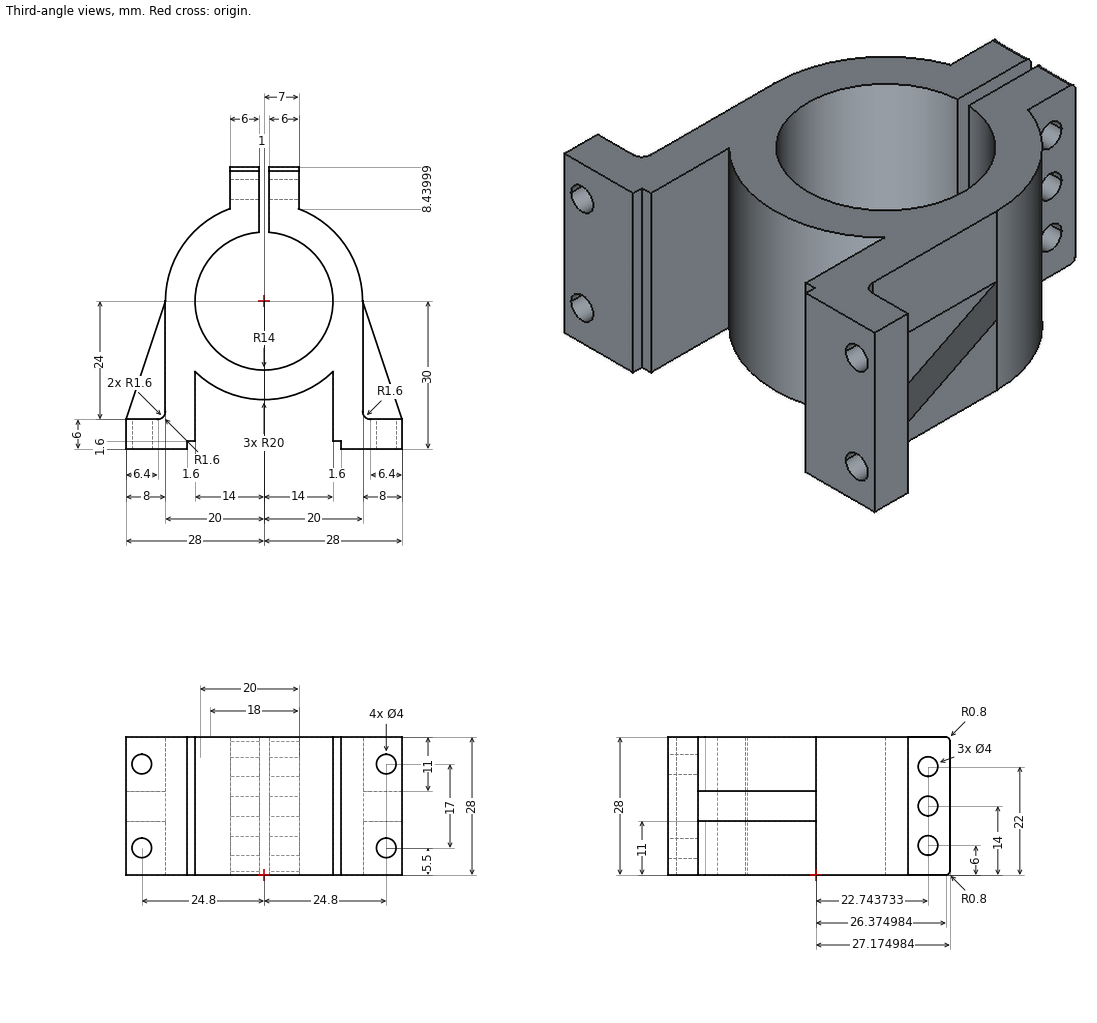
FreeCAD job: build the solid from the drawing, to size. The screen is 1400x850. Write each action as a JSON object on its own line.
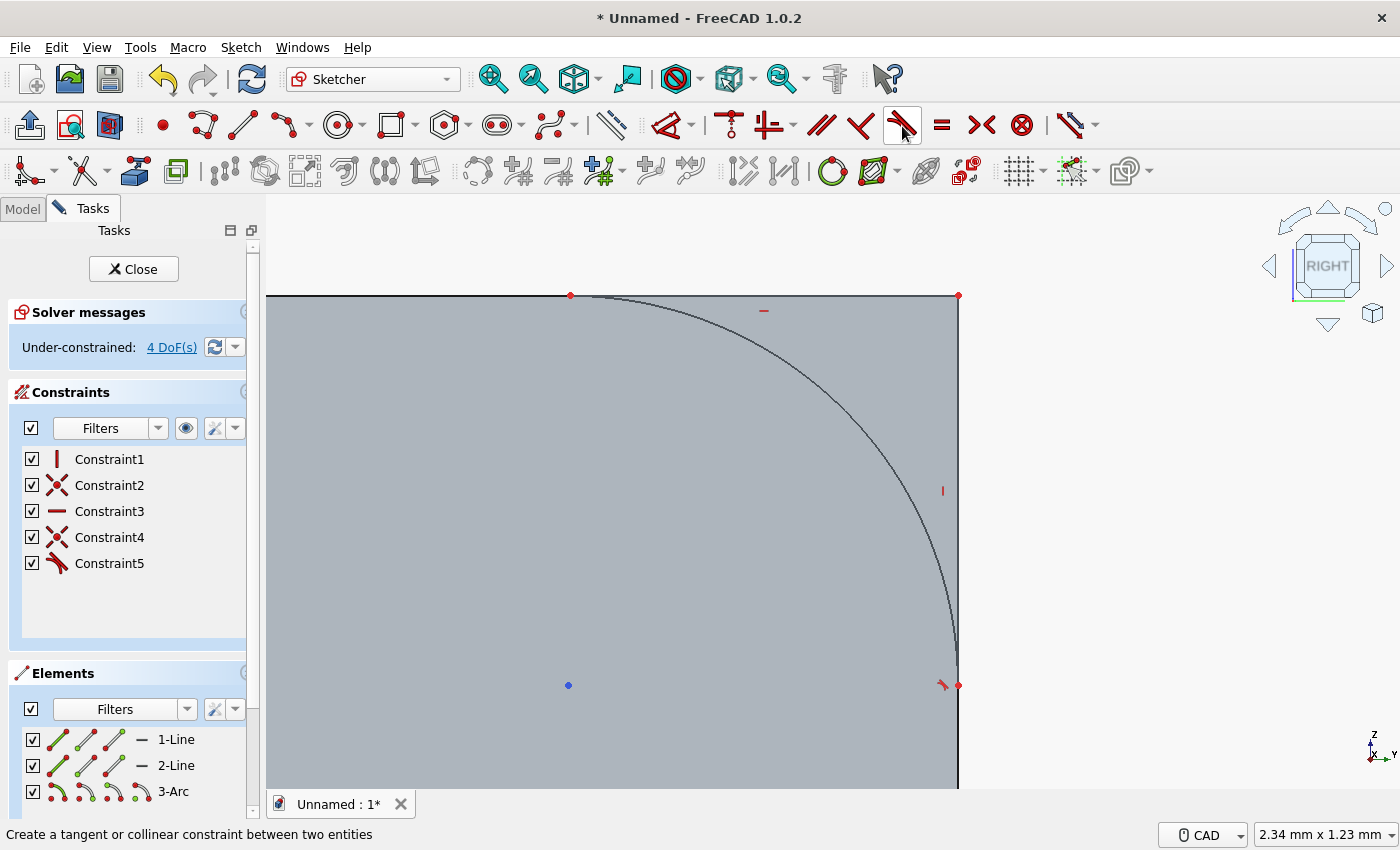
{"action": "left_click", "coordinate": [842, 296]}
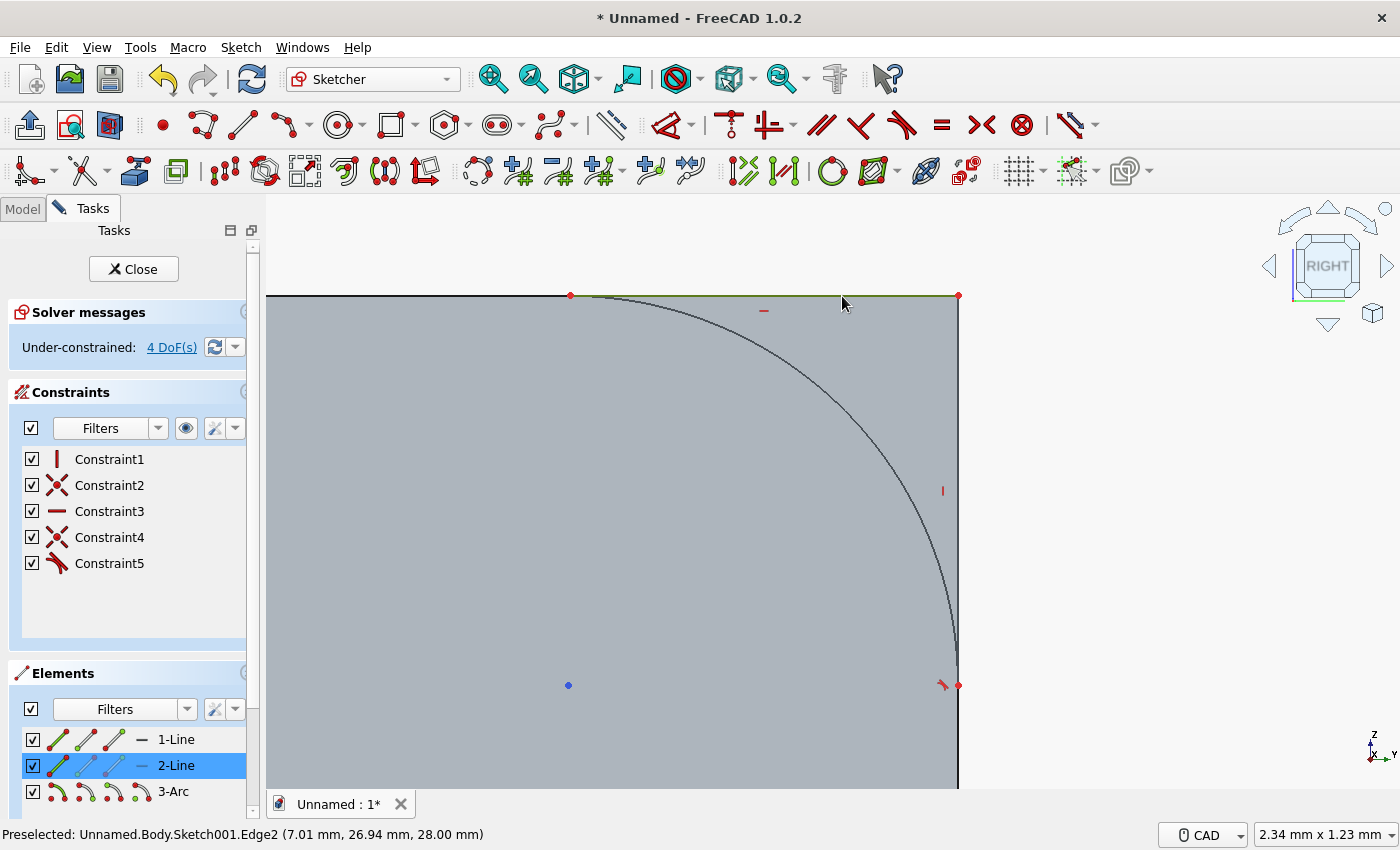
{"action": "left_click", "coordinate": [916, 509]}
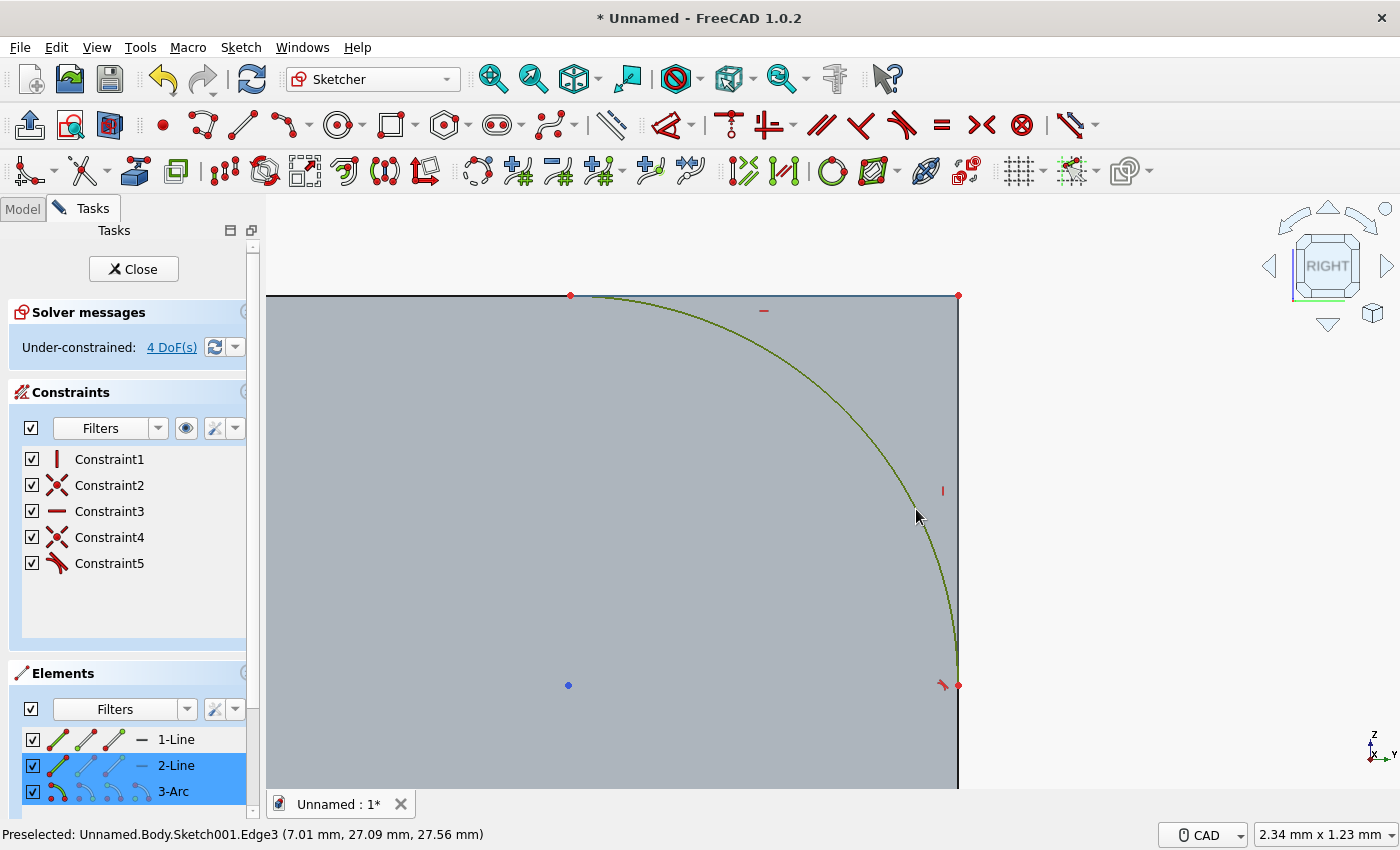
{"action": "left_click", "coordinate": [902, 126]}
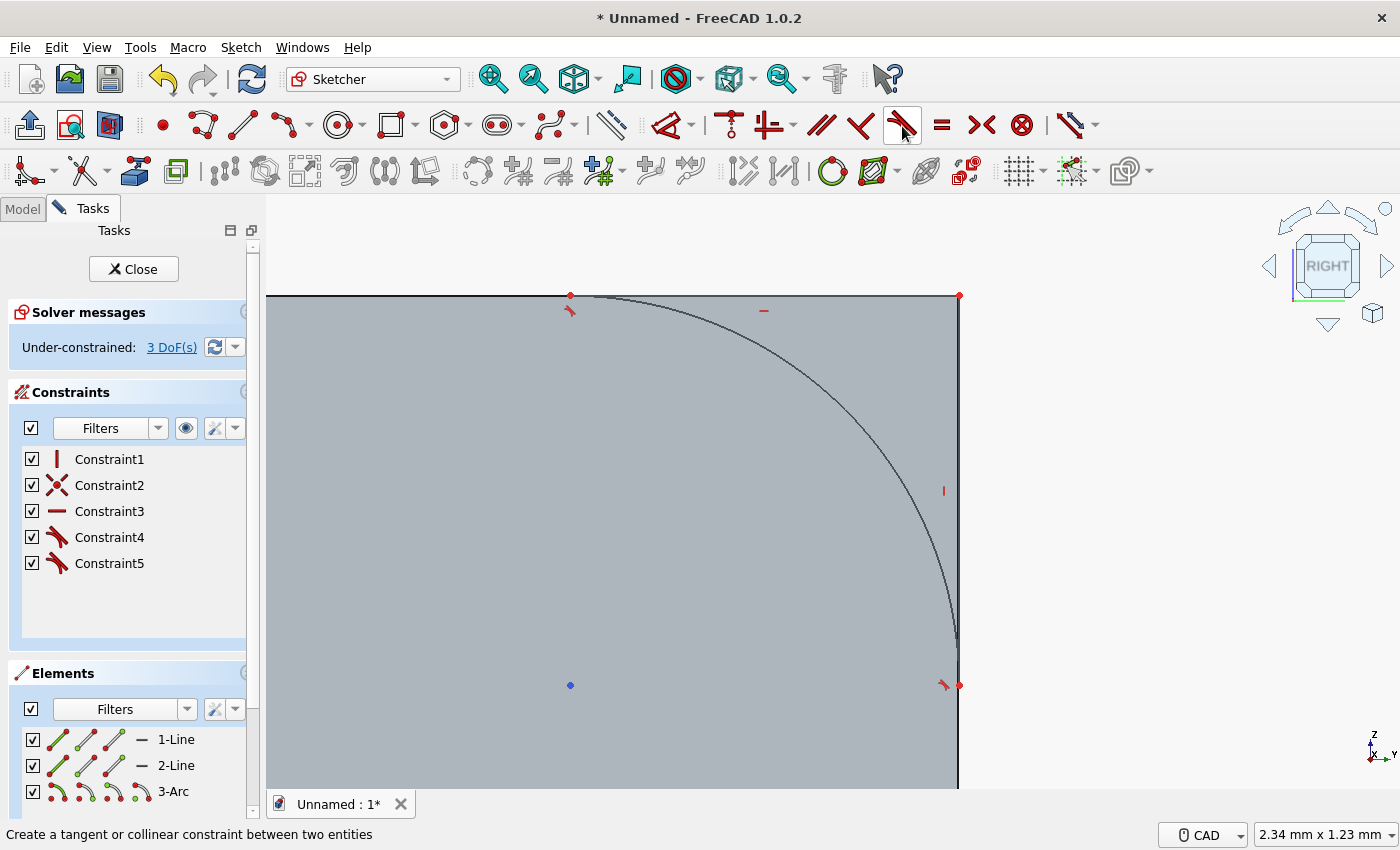
{"action": "left_click", "coordinate": [666, 126]}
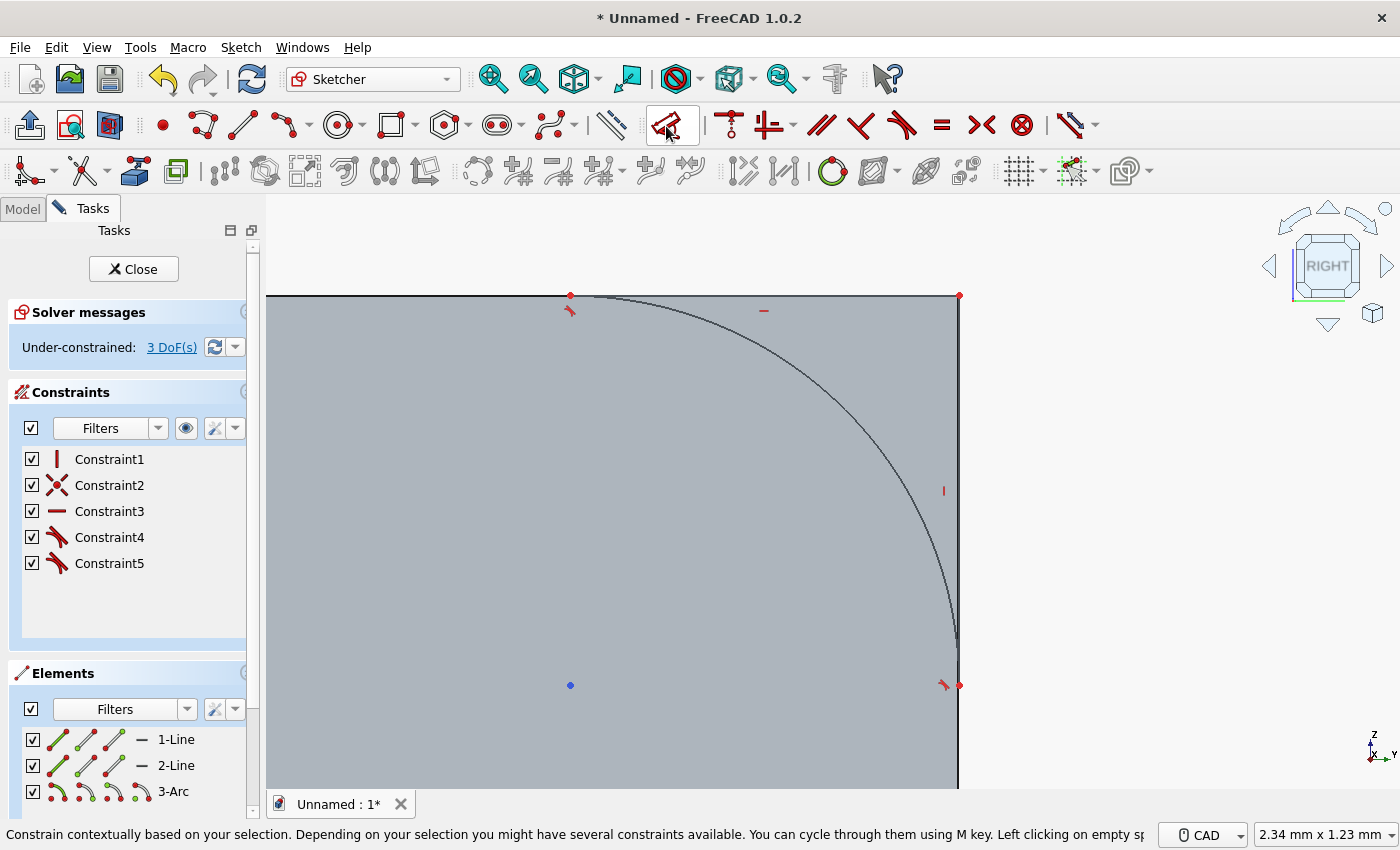
{"action": "left_click", "coordinate": [917, 508]}
{"action": "left_click", "coordinate": [946, 493]}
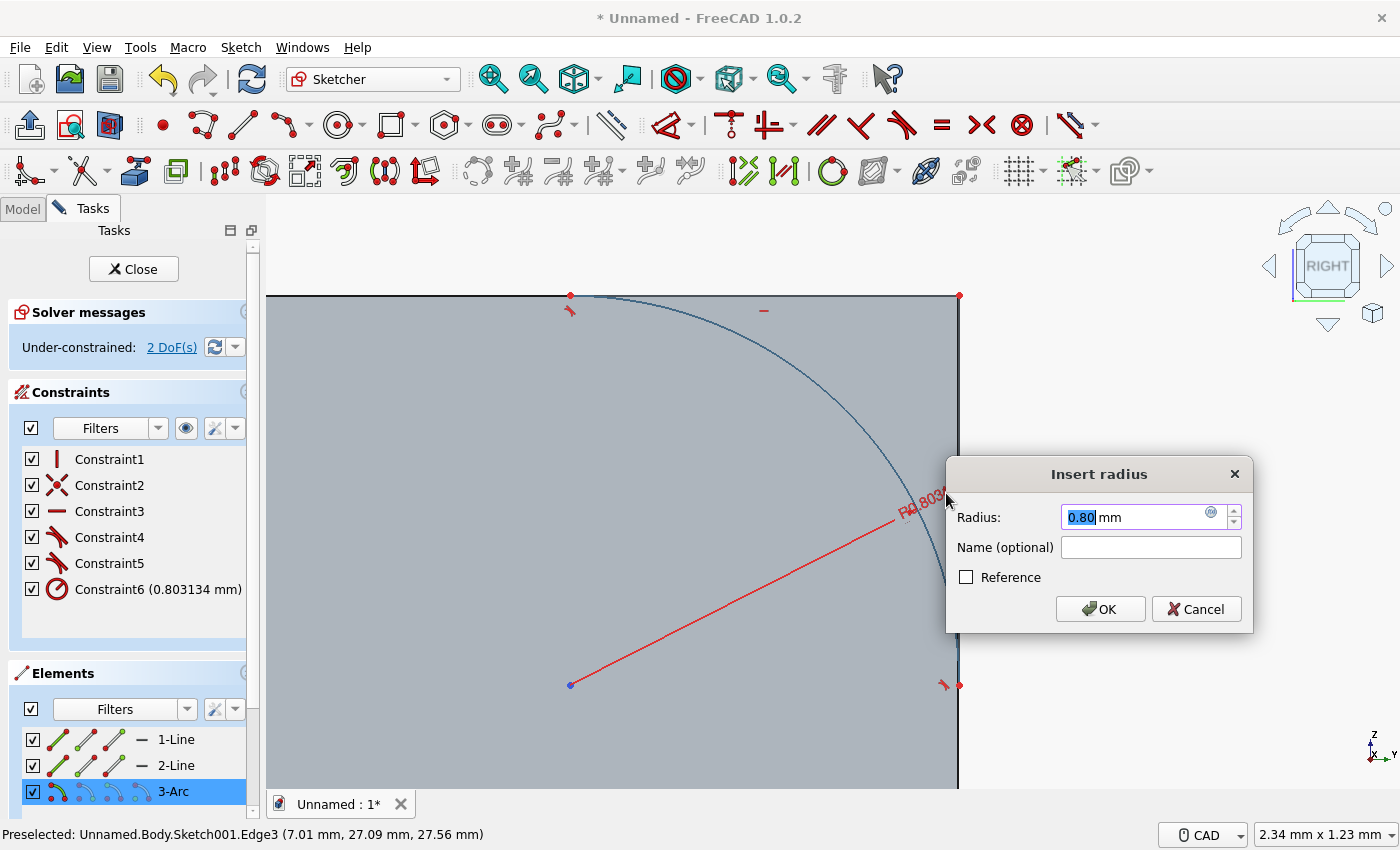
{"action": "type", "text": "0.8"}
{"action": "key", "text": "Return"}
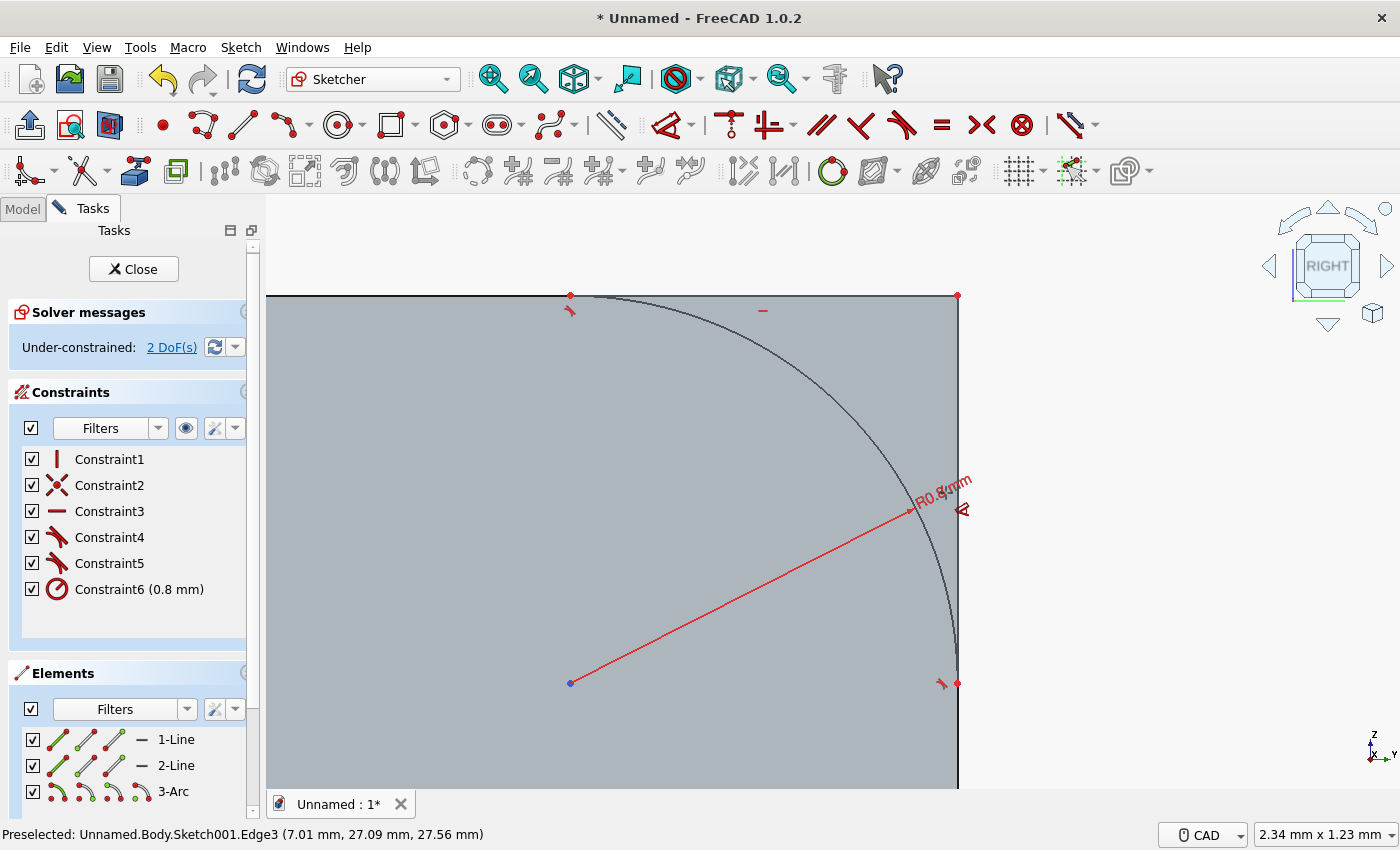
{"action": "left_click", "coordinate": [958, 296]}
{"action": "left_click", "coordinate": [992, 528]}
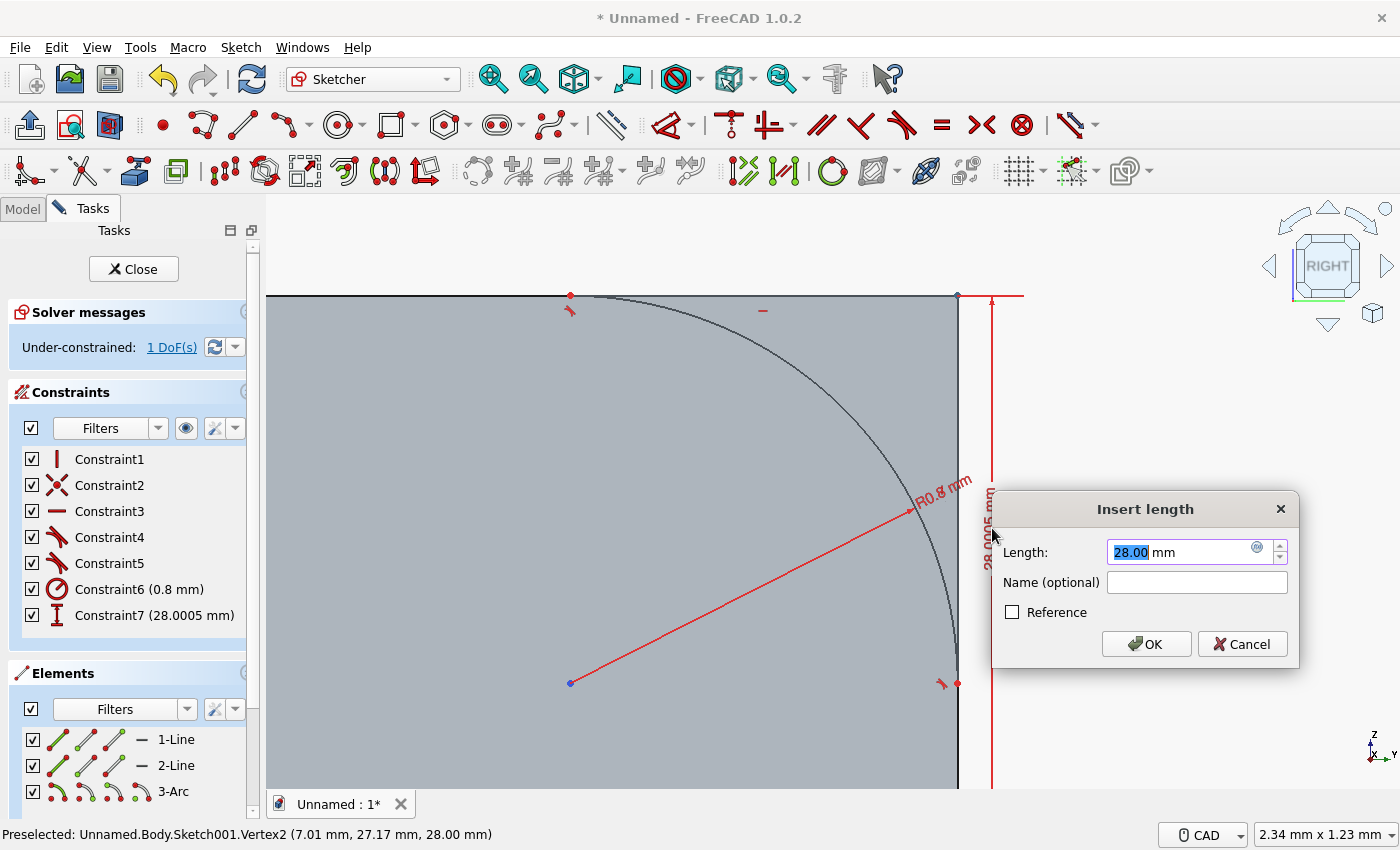
{"action": "type", "text": "28"}
{"action": "key", "text": "Return"}